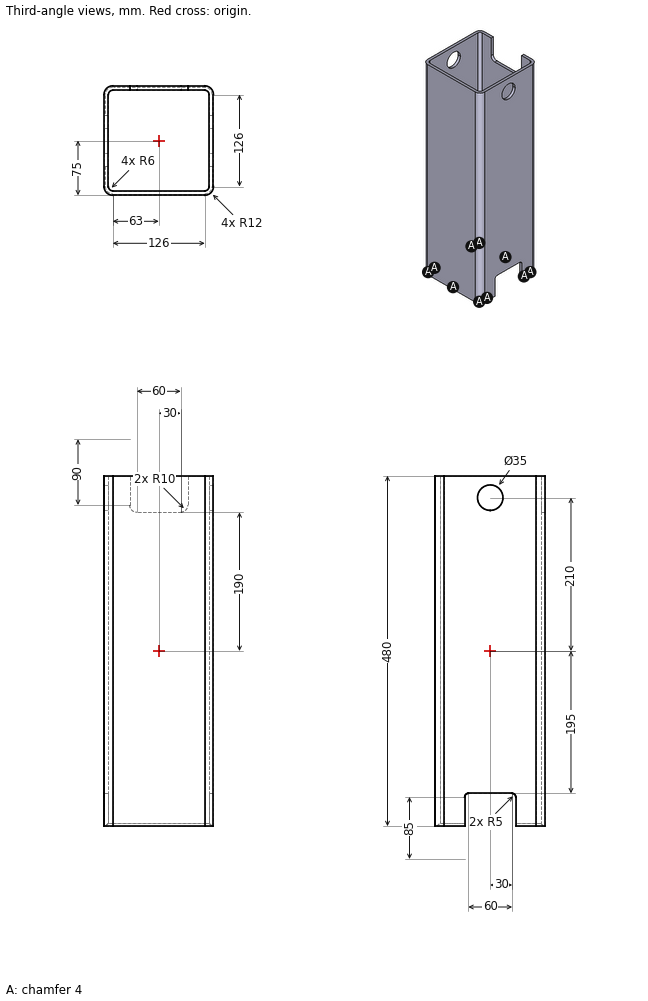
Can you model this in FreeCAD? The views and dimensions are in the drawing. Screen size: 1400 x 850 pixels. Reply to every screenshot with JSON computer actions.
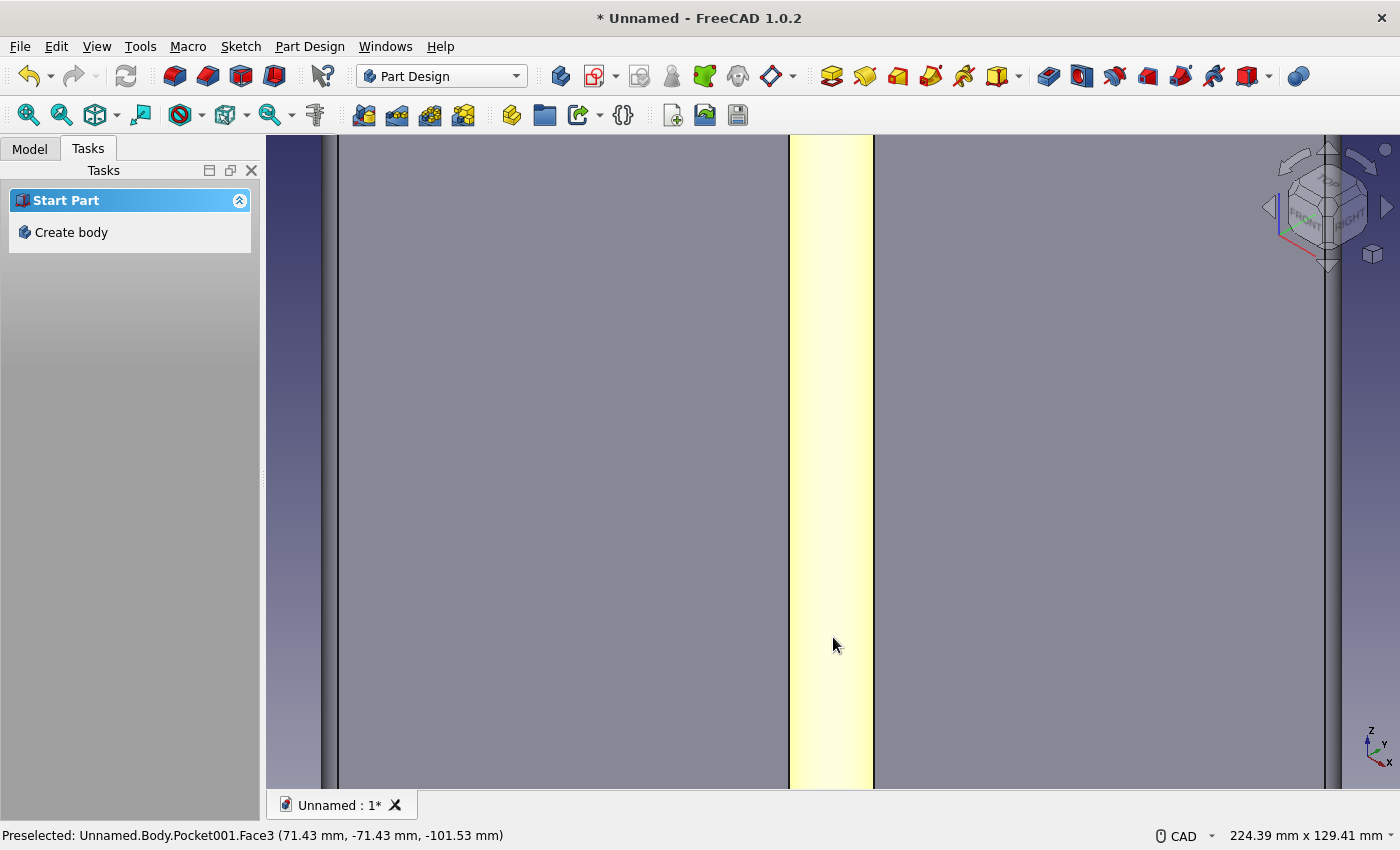
{"action": "key", "text": "v f"}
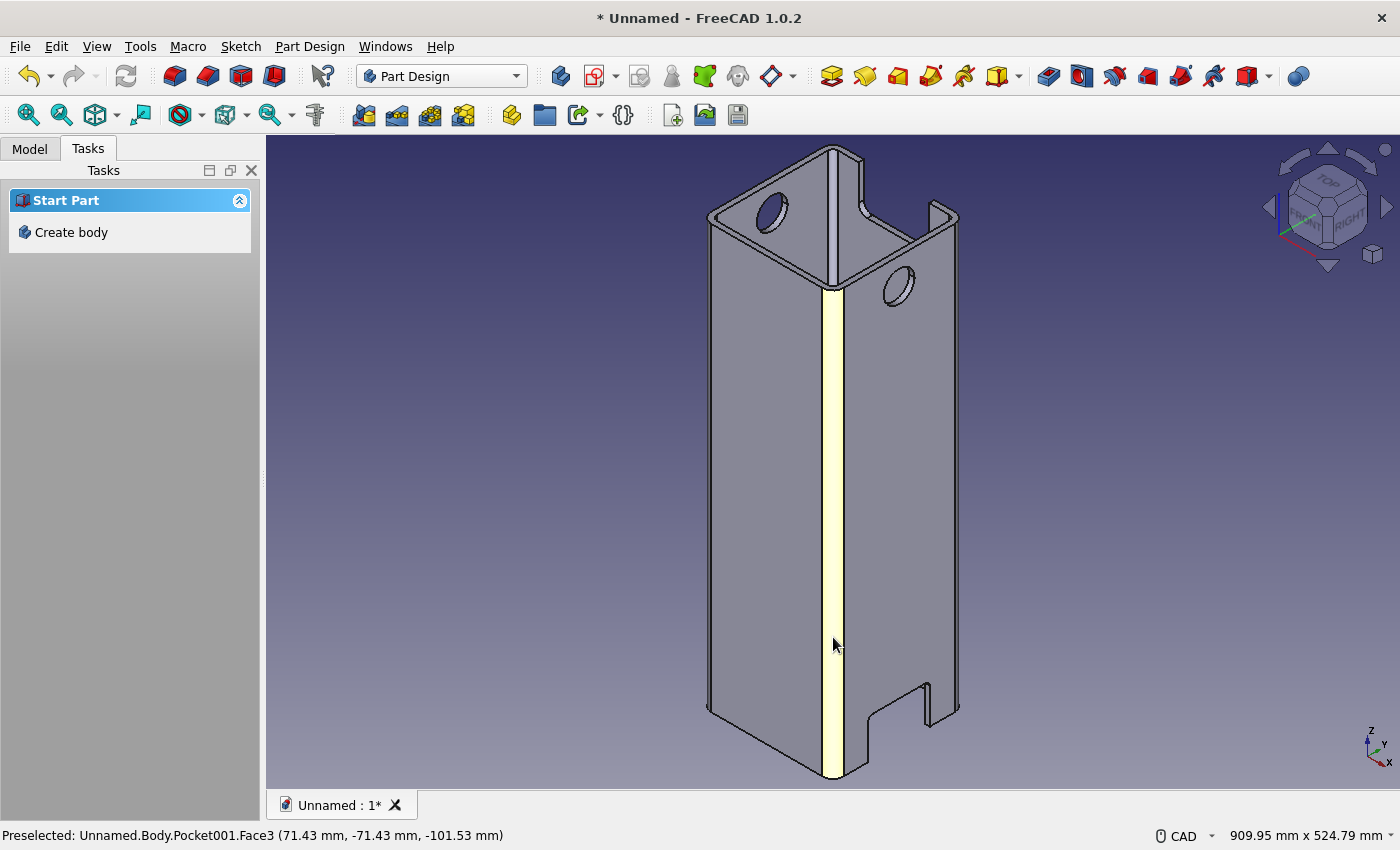
{"action": "key", "text": "2"}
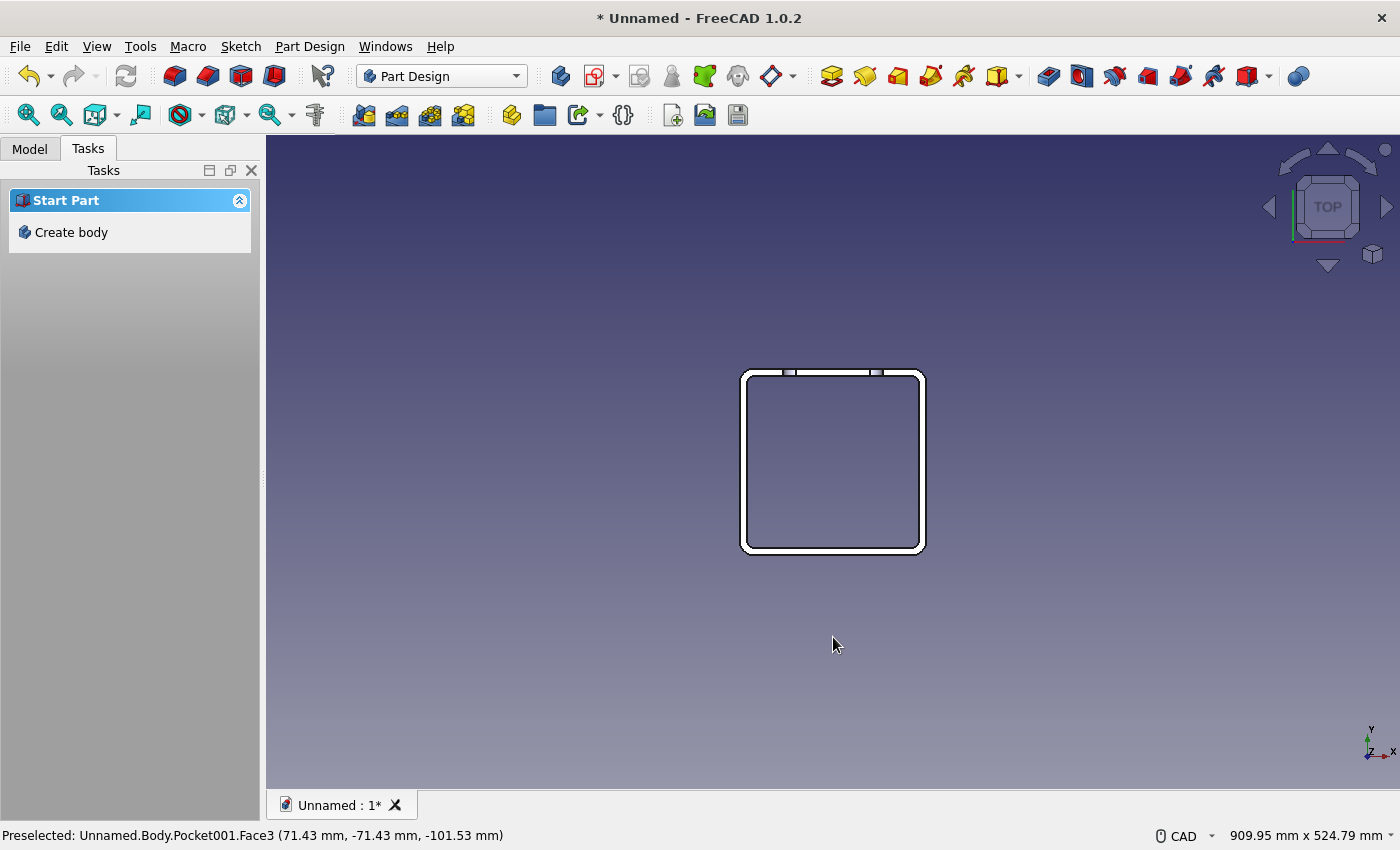
{"action": "key", "text": "v f"}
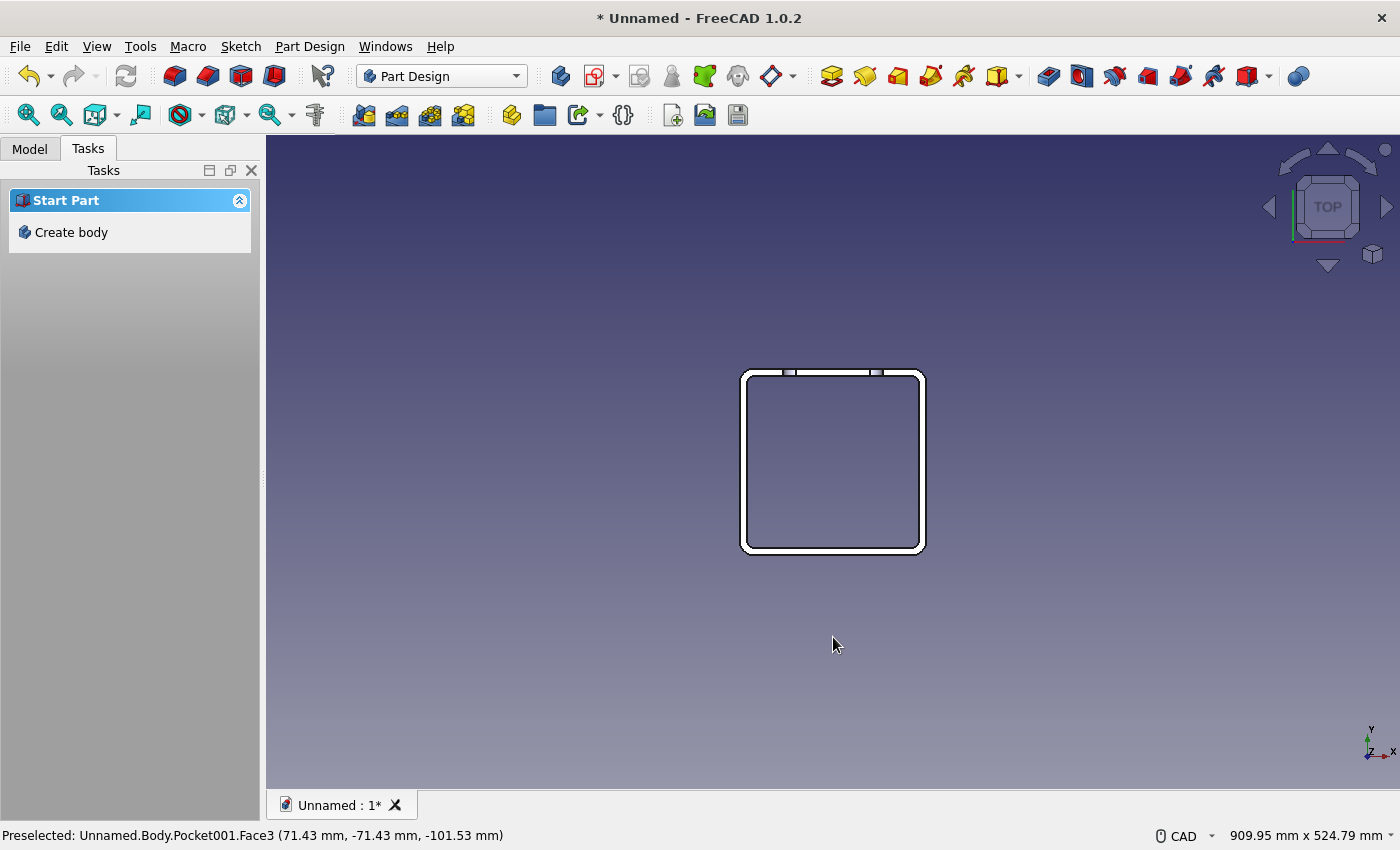
{"action": "scroll", "coordinate": [749, 377], "scroll_direction": "up", "scroll_amount": 7}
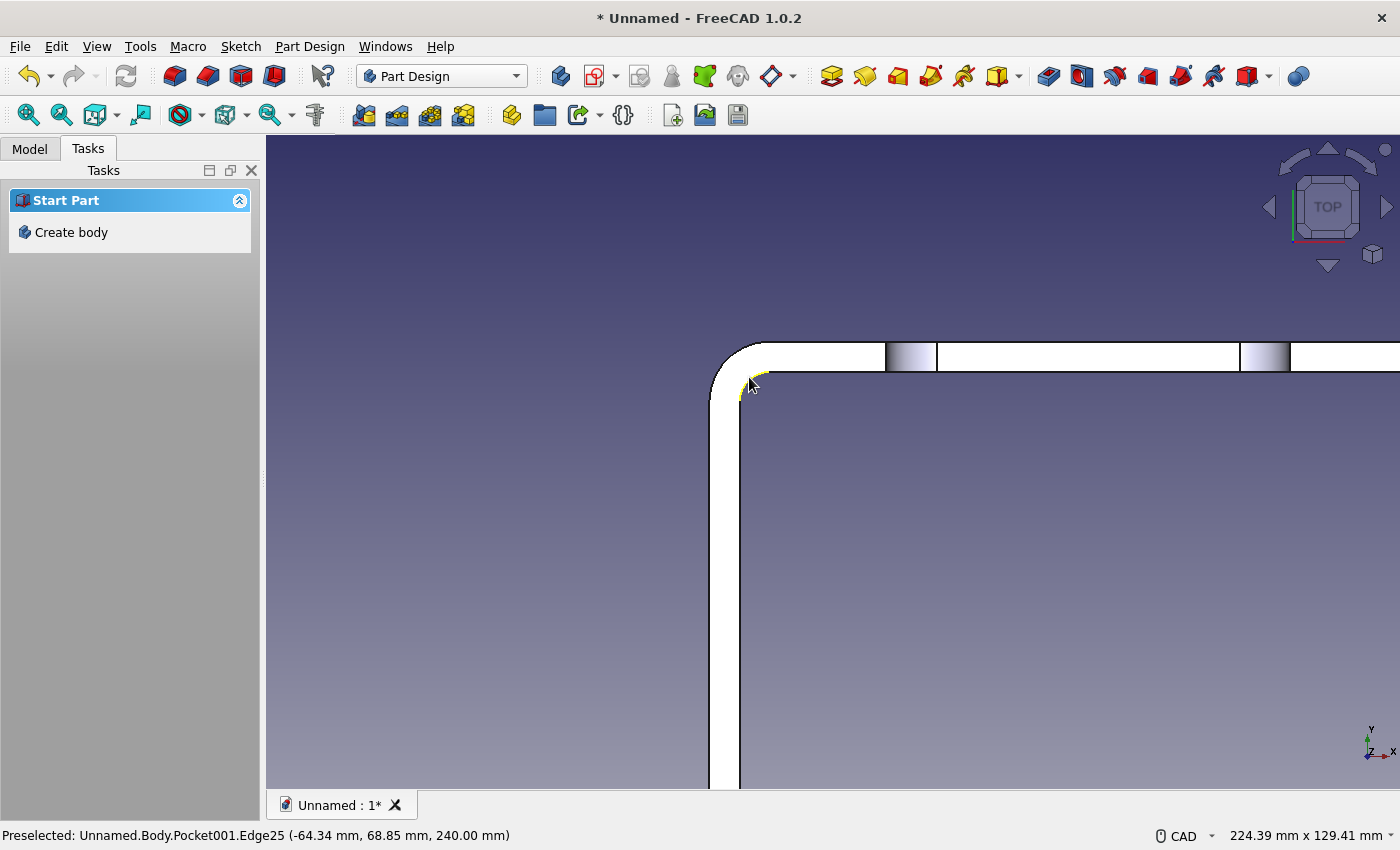
{"action": "key", "text": "v f"}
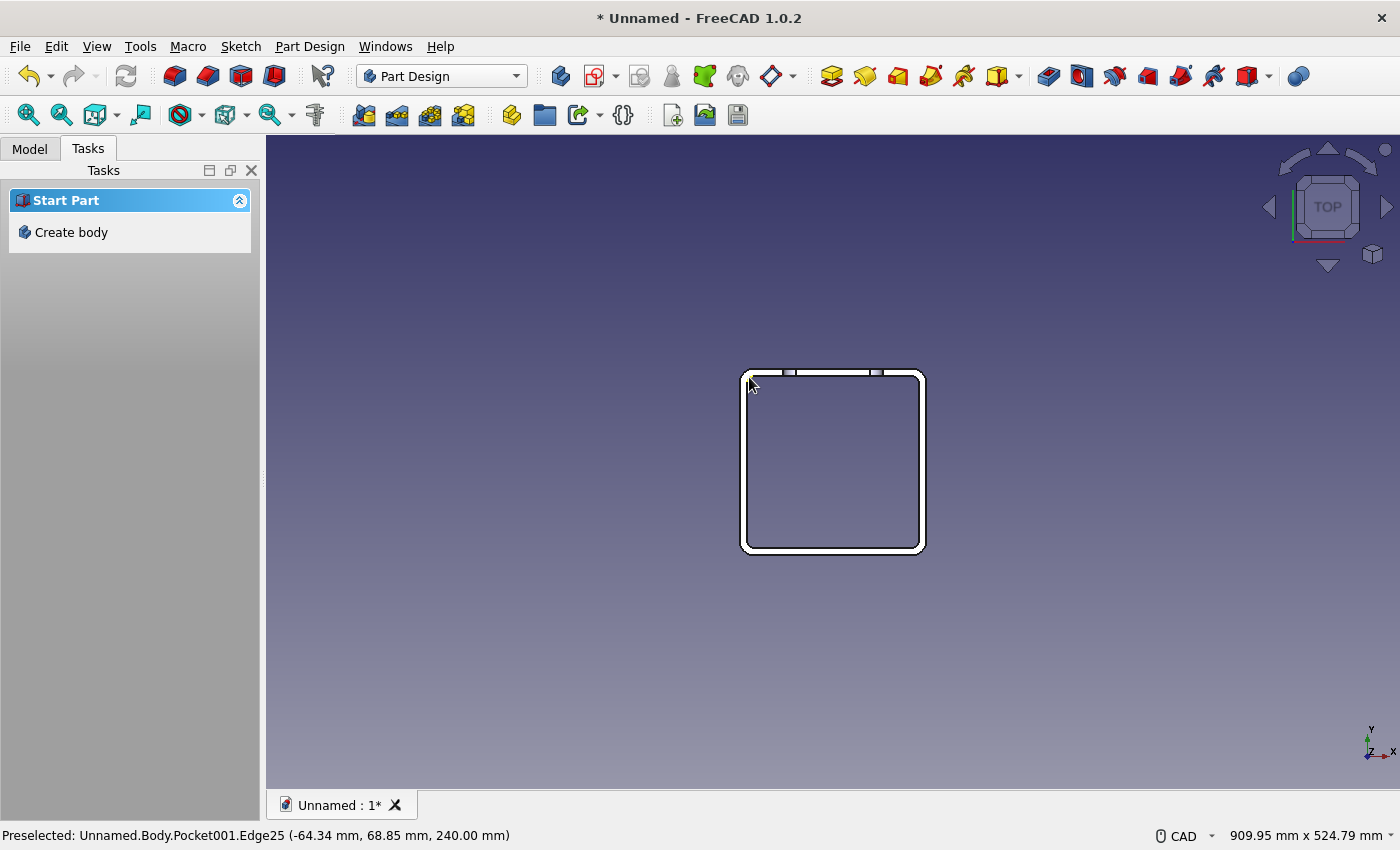
{"action": "key", "text": "1"}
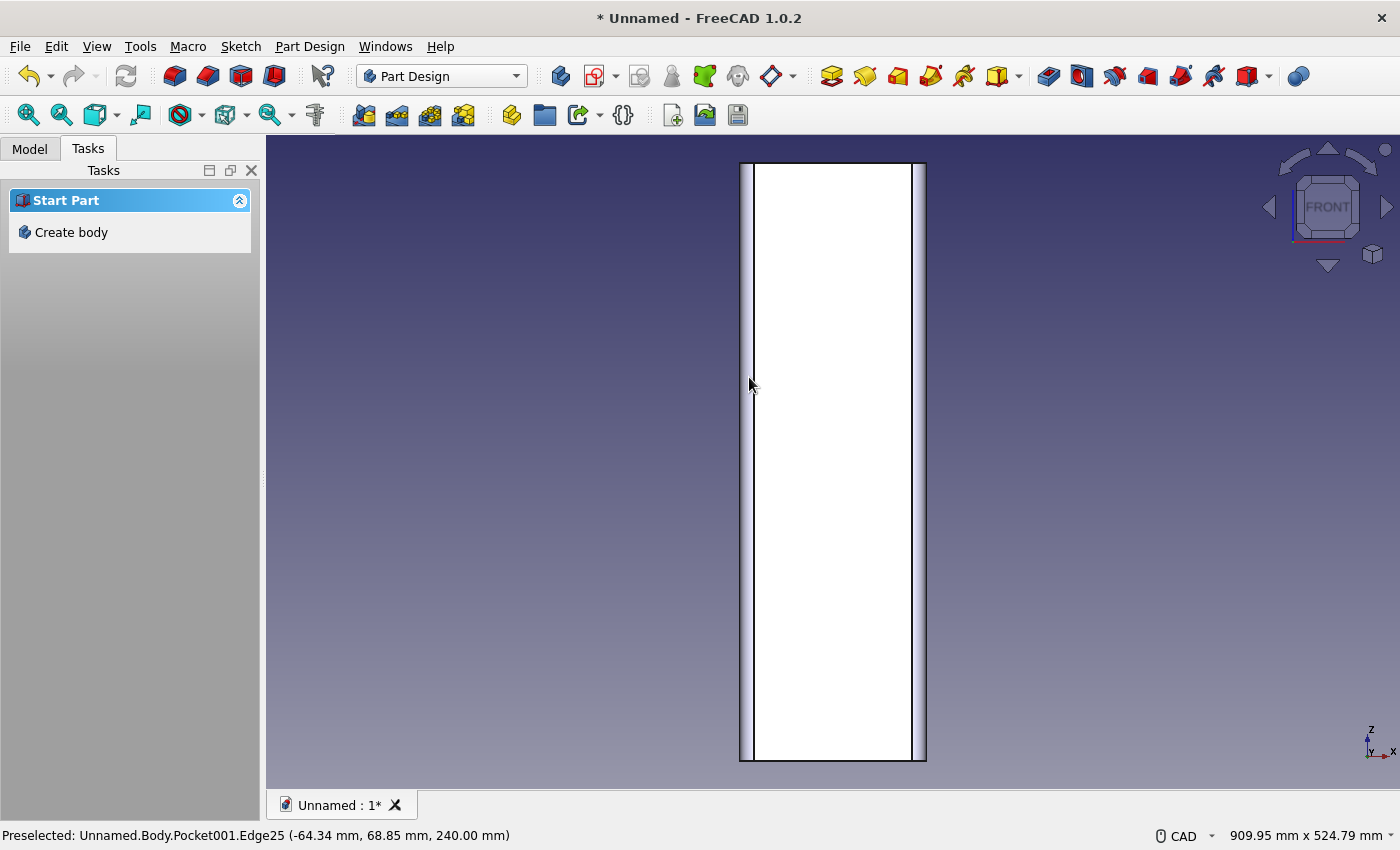
{"action": "scroll", "coordinate": [749, 760], "scroll_direction": "up", "scroll_amount": 7}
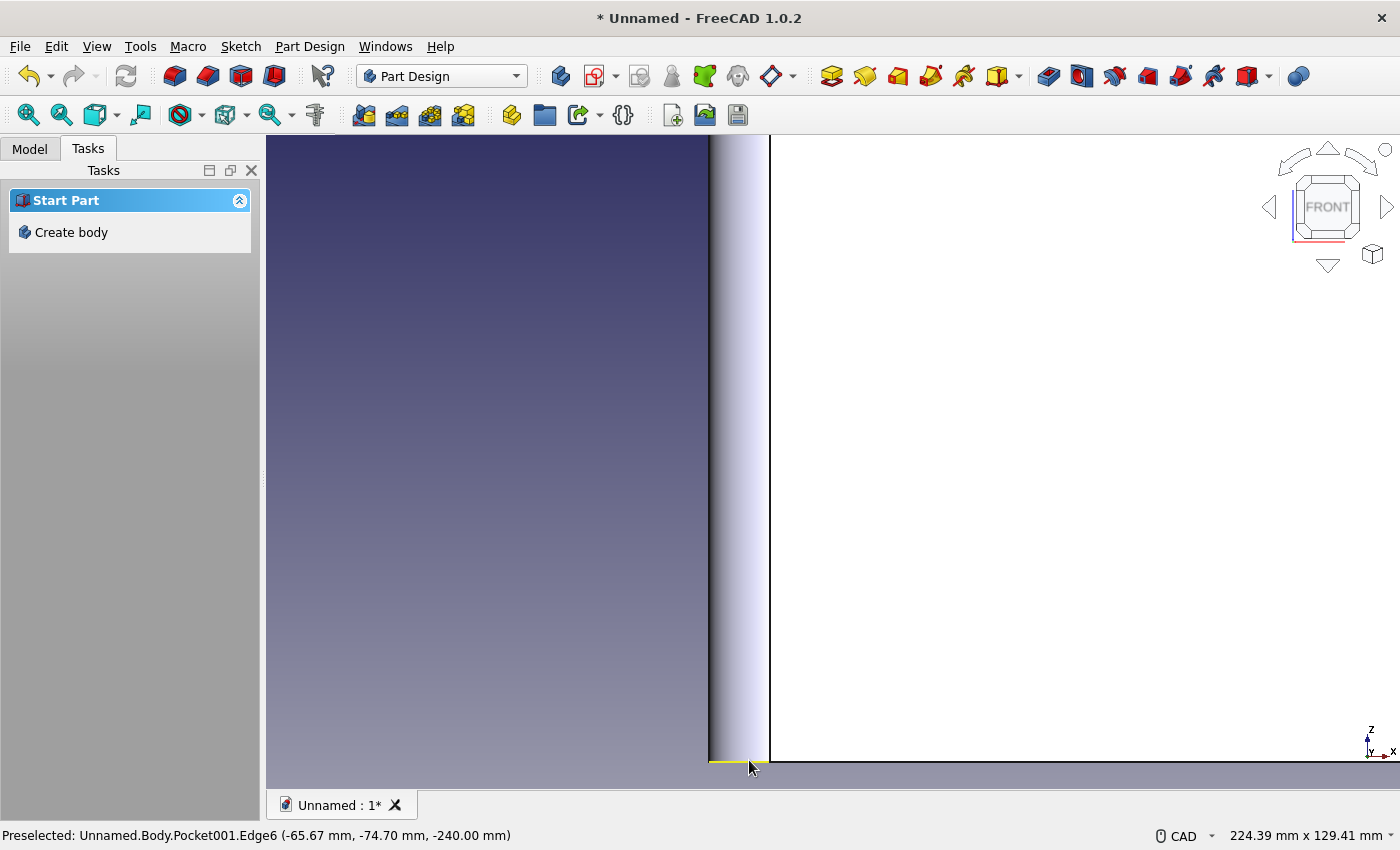
{"action": "key", "text": "v f"}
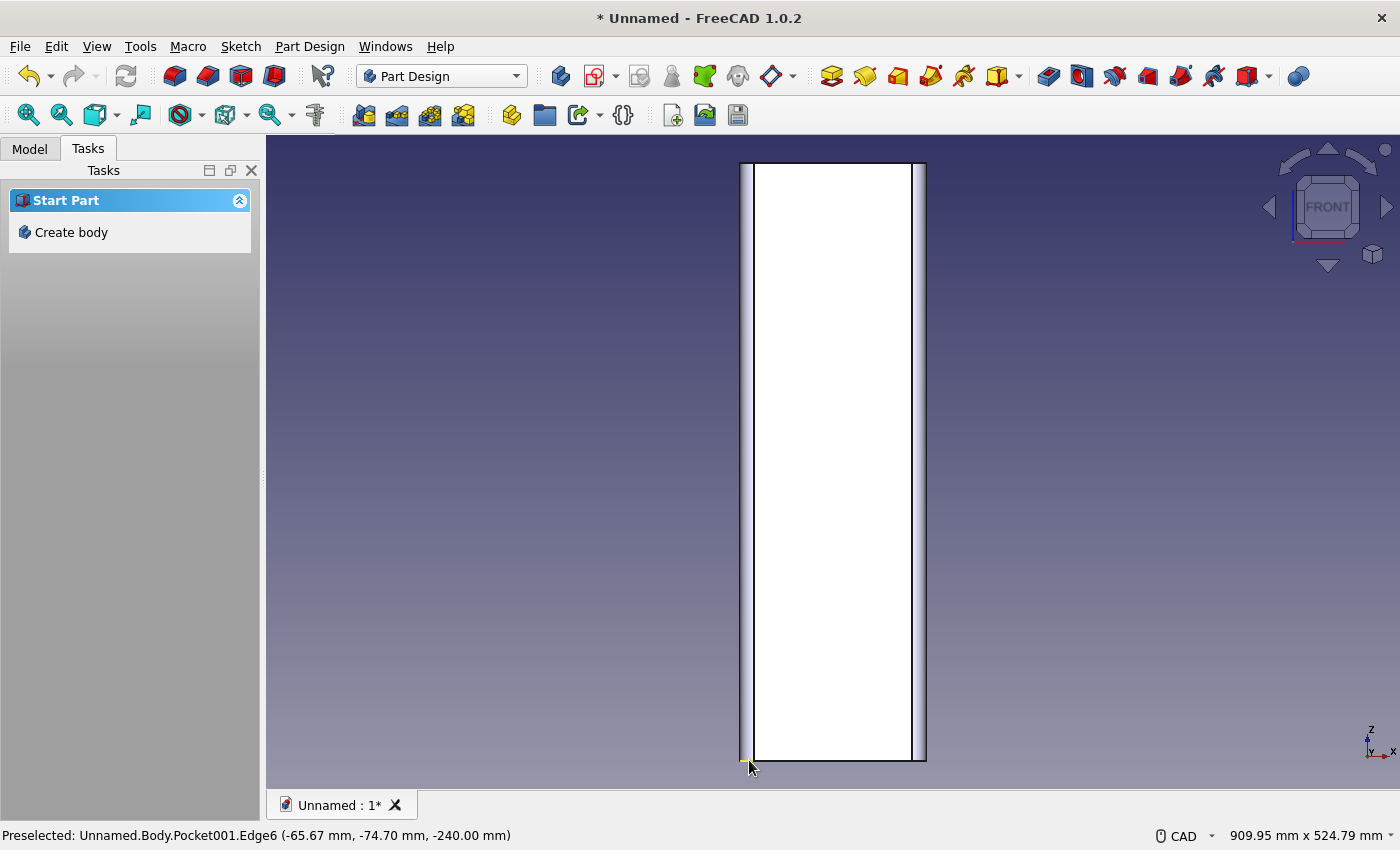
{"action": "key", "text": "3"}